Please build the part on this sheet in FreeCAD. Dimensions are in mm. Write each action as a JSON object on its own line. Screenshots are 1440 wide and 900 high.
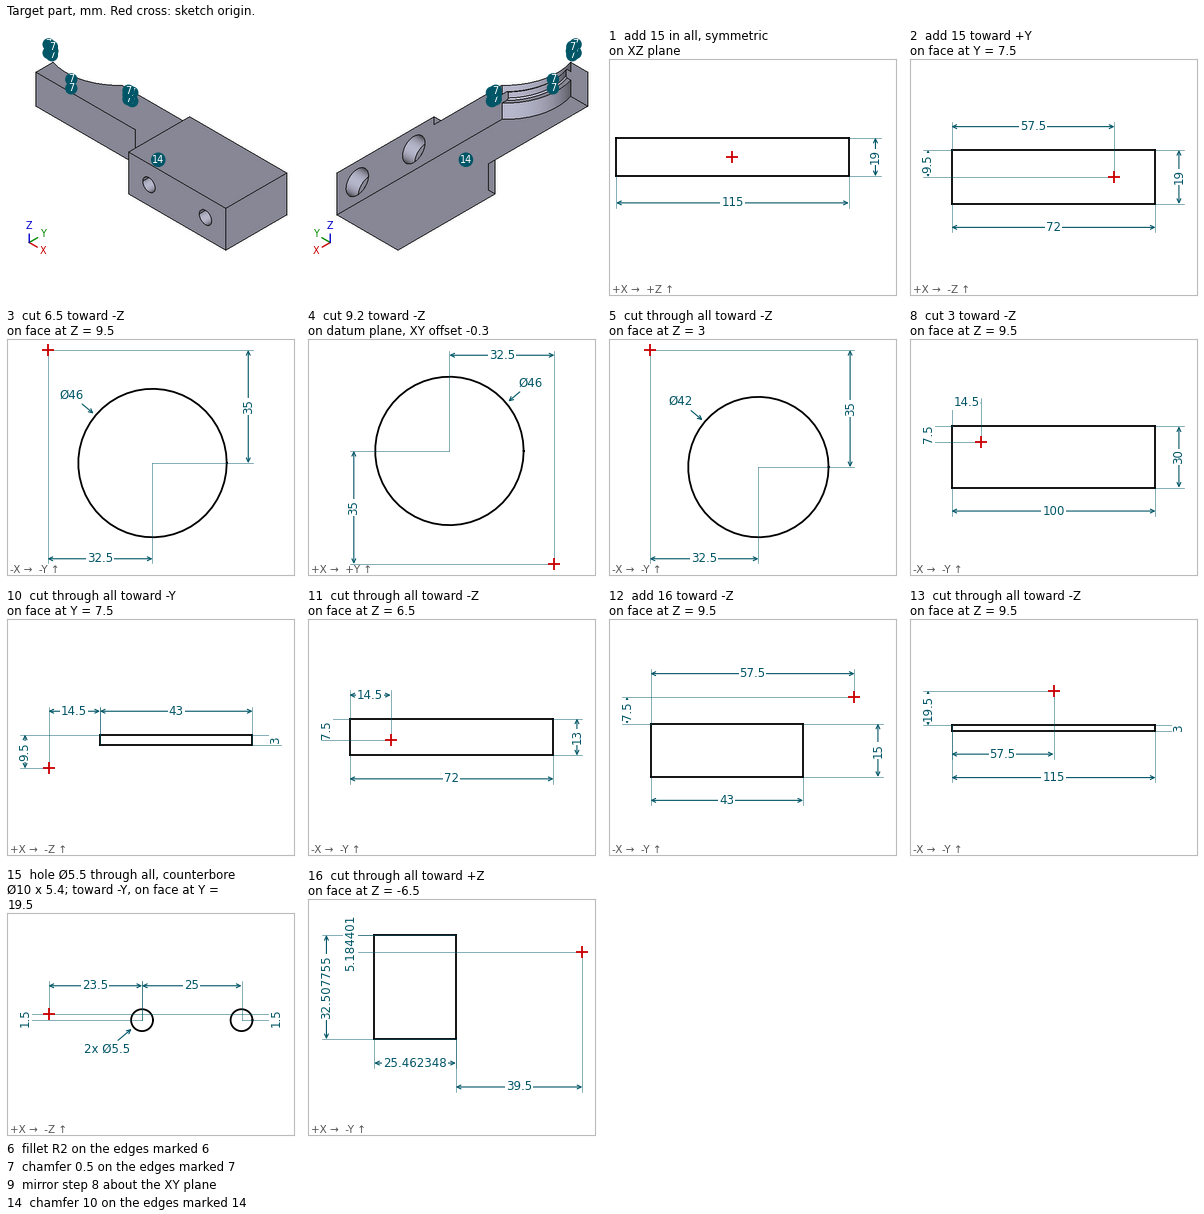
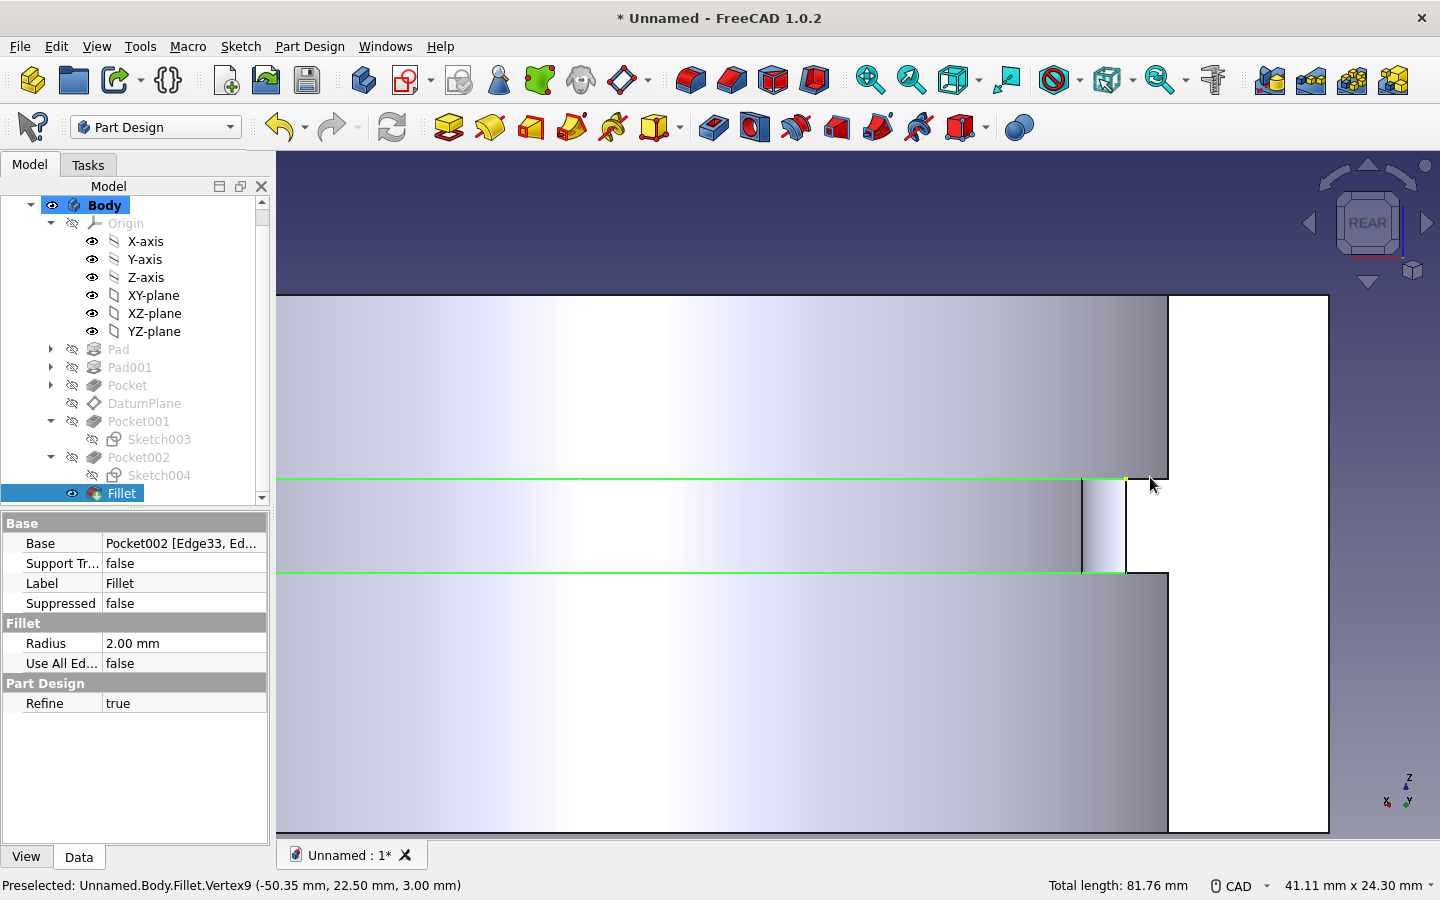
{"action": "left_click", "coordinate": [1147, 572], "text": "ctrl"}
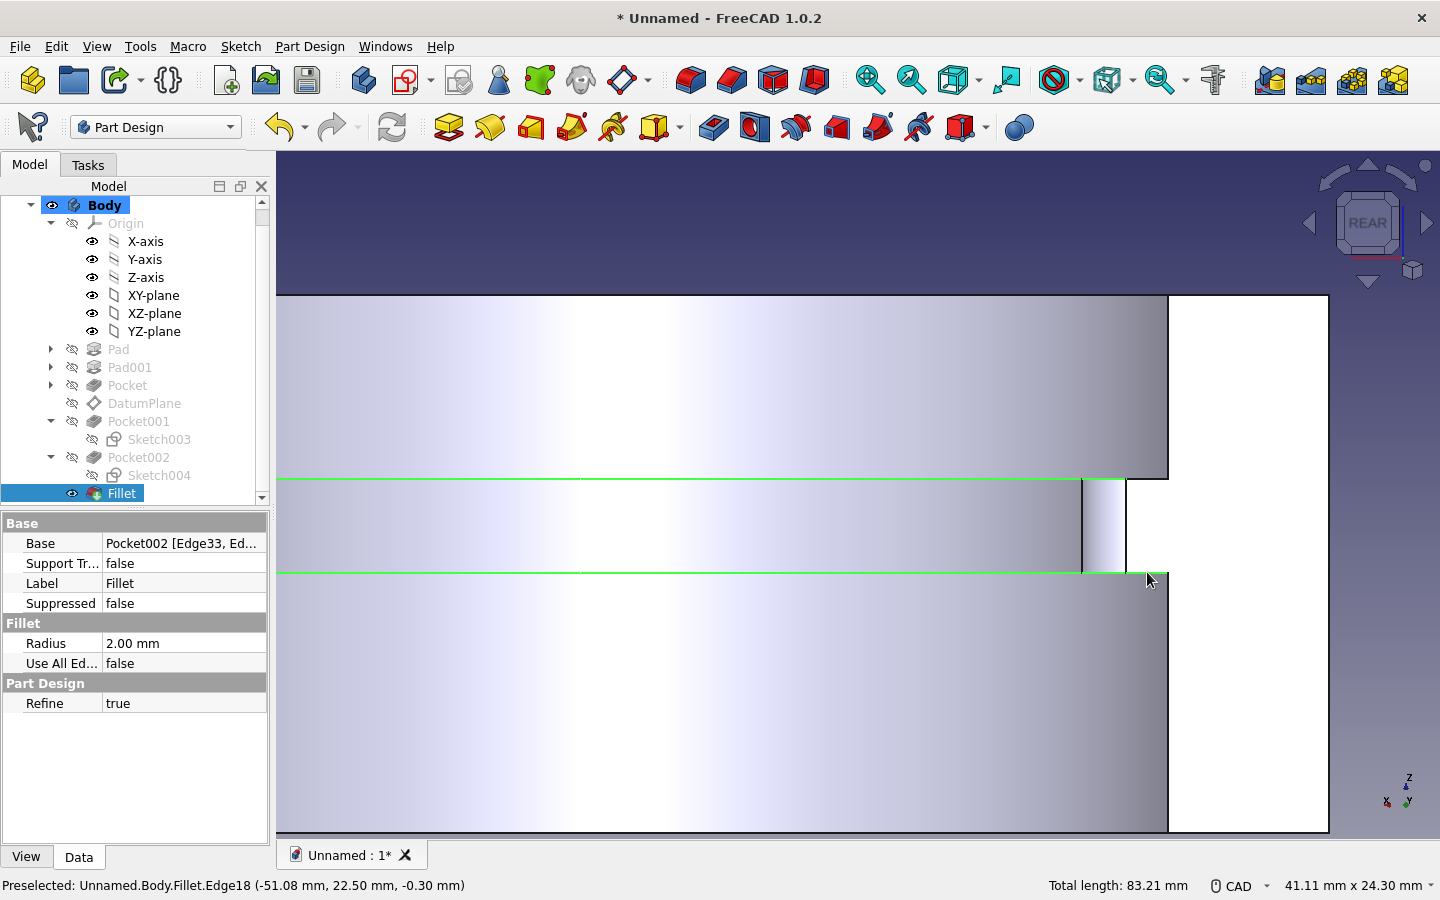
{"action": "left_click", "coordinate": [871, 80]}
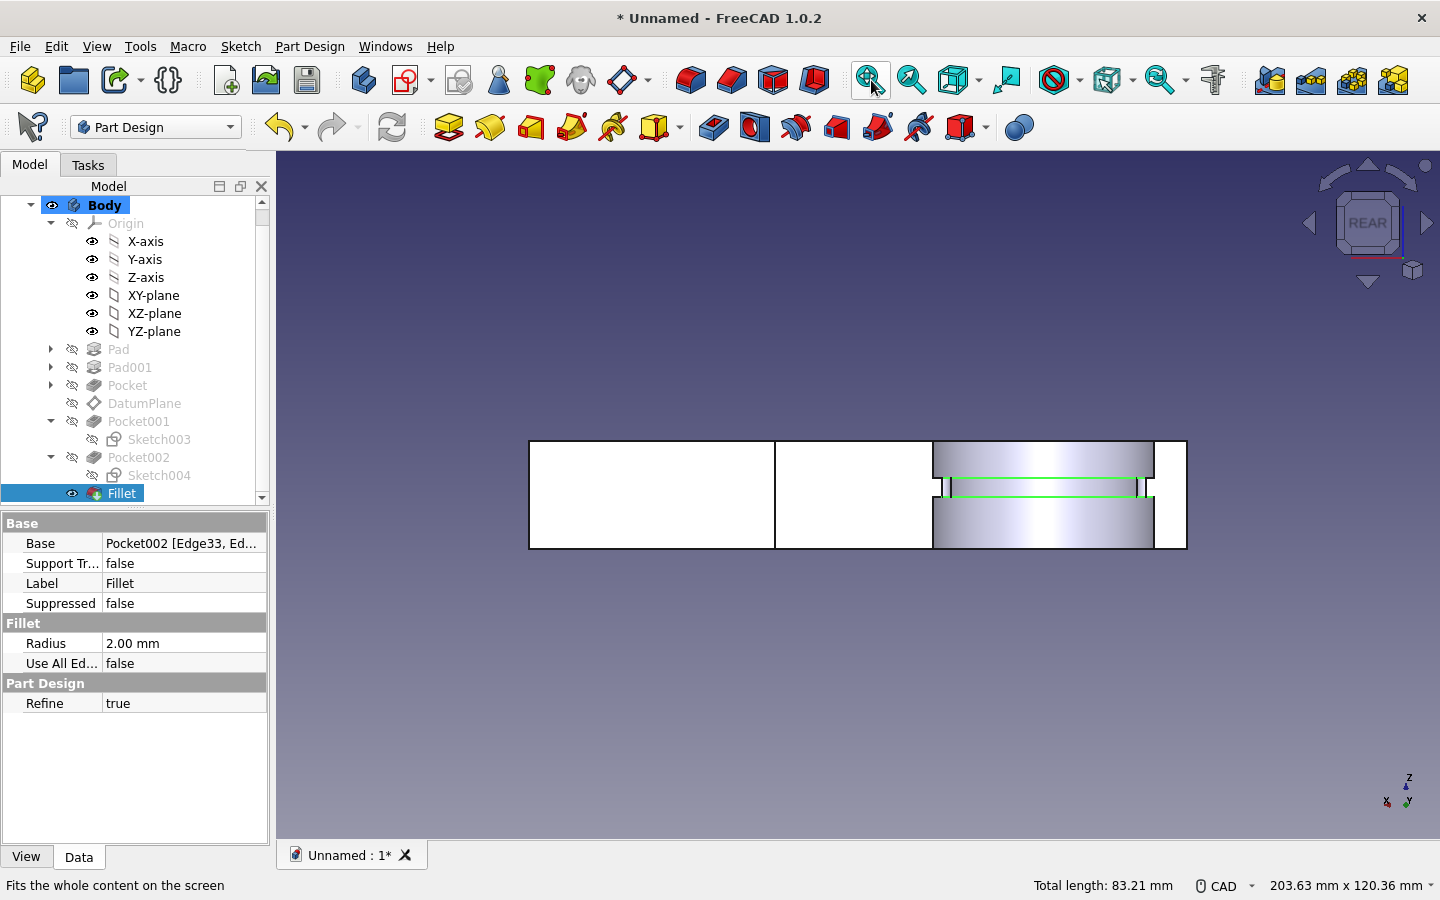
{"action": "key", "text": "0"}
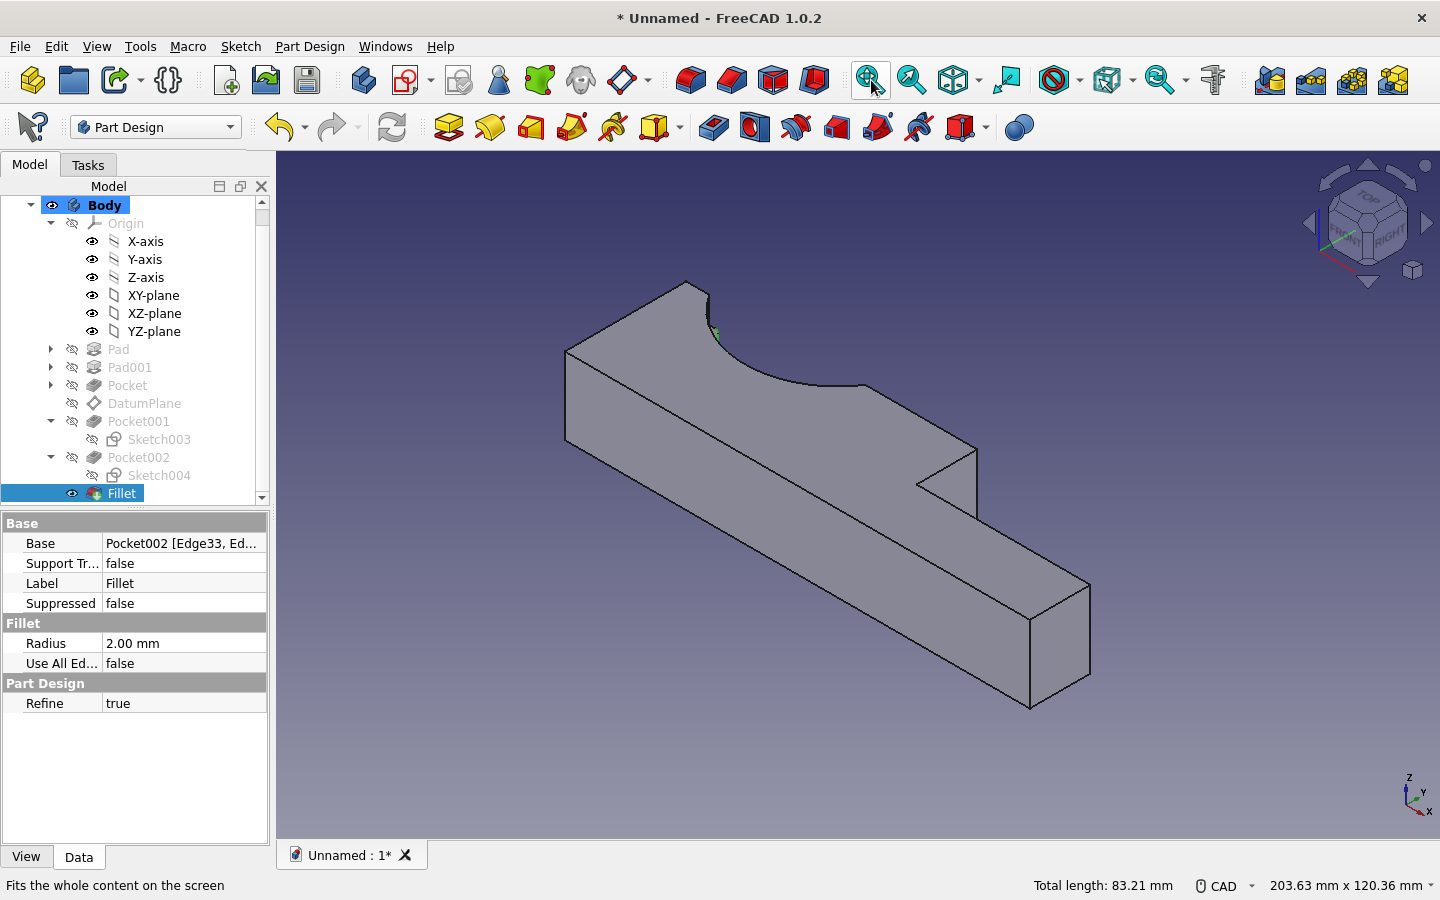
{"action": "scroll", "coordinate": [712, 326], "scroll_direction": "up", "scroll_amount": 8}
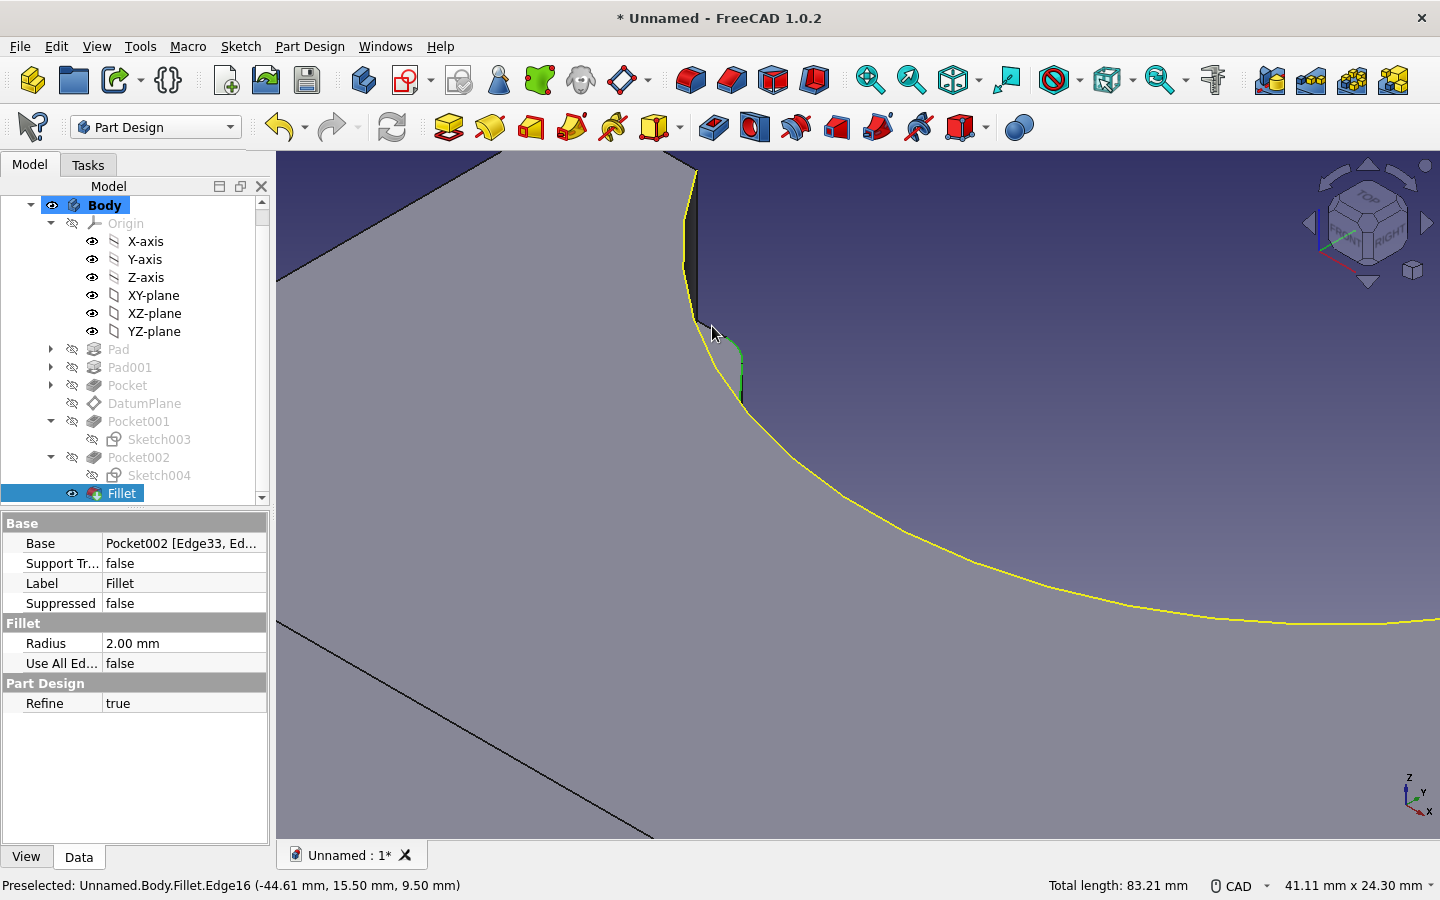
{"action": "left_click", "coordinate": [871, 80]}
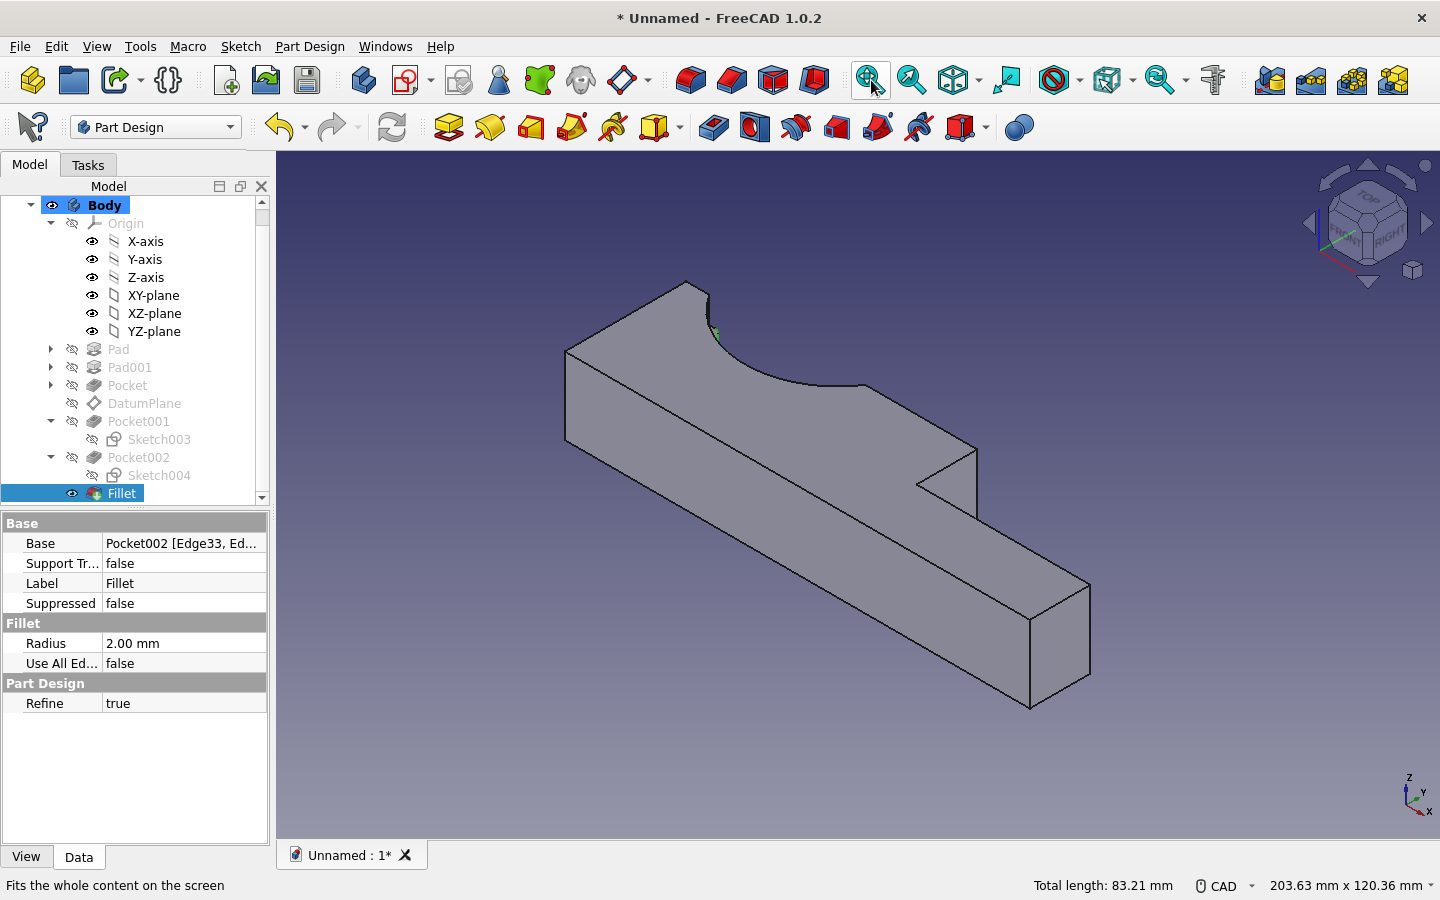
{"action": "key", "text": "2"}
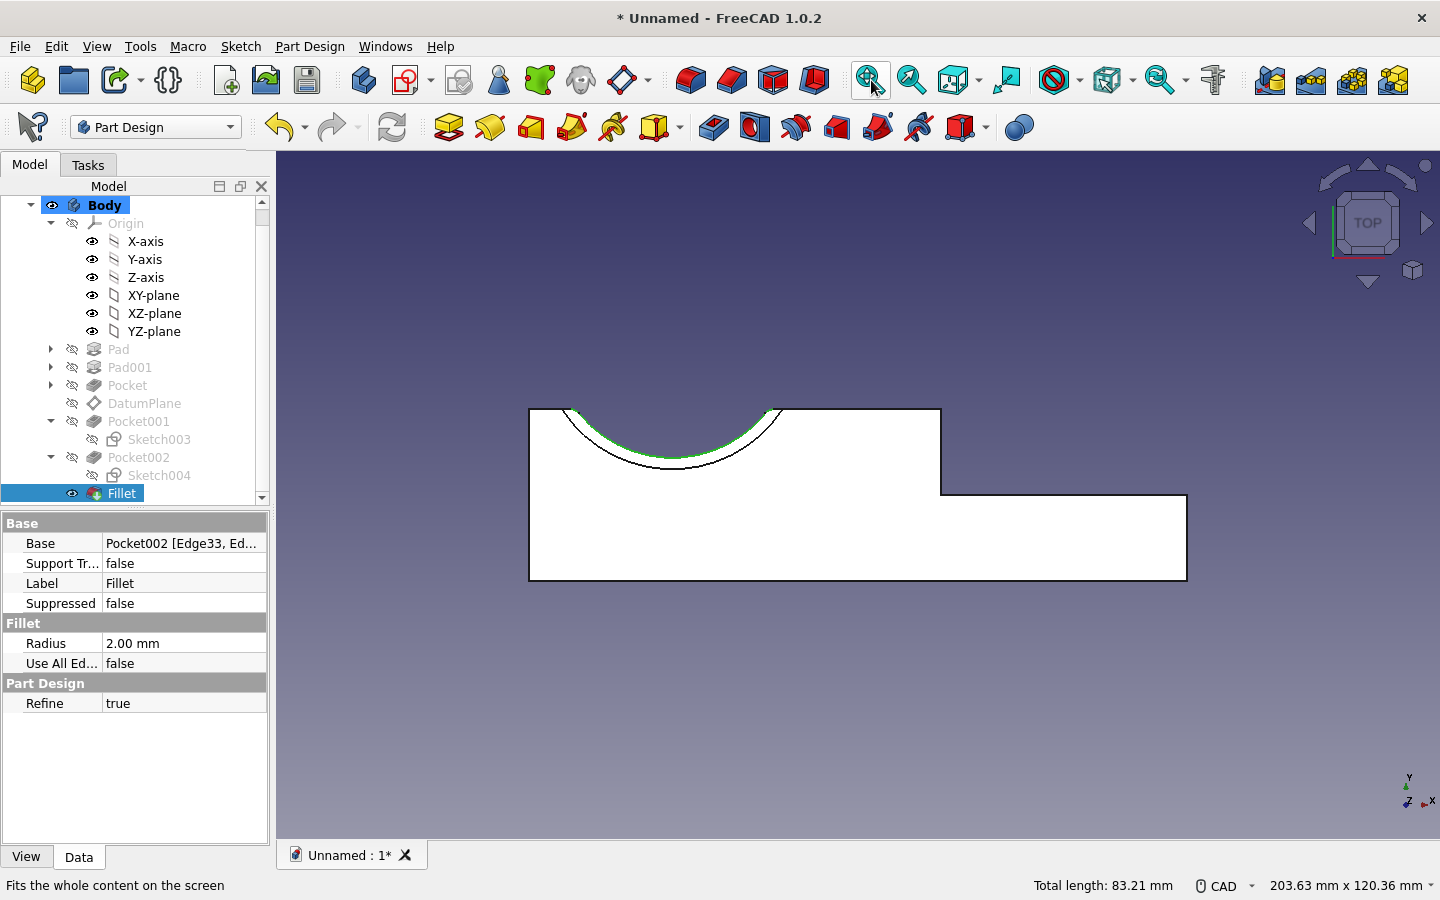
{"action": "scroll", "coordinate": [566, 408], "scroll_direction": "up", "scroll_amount": 8}